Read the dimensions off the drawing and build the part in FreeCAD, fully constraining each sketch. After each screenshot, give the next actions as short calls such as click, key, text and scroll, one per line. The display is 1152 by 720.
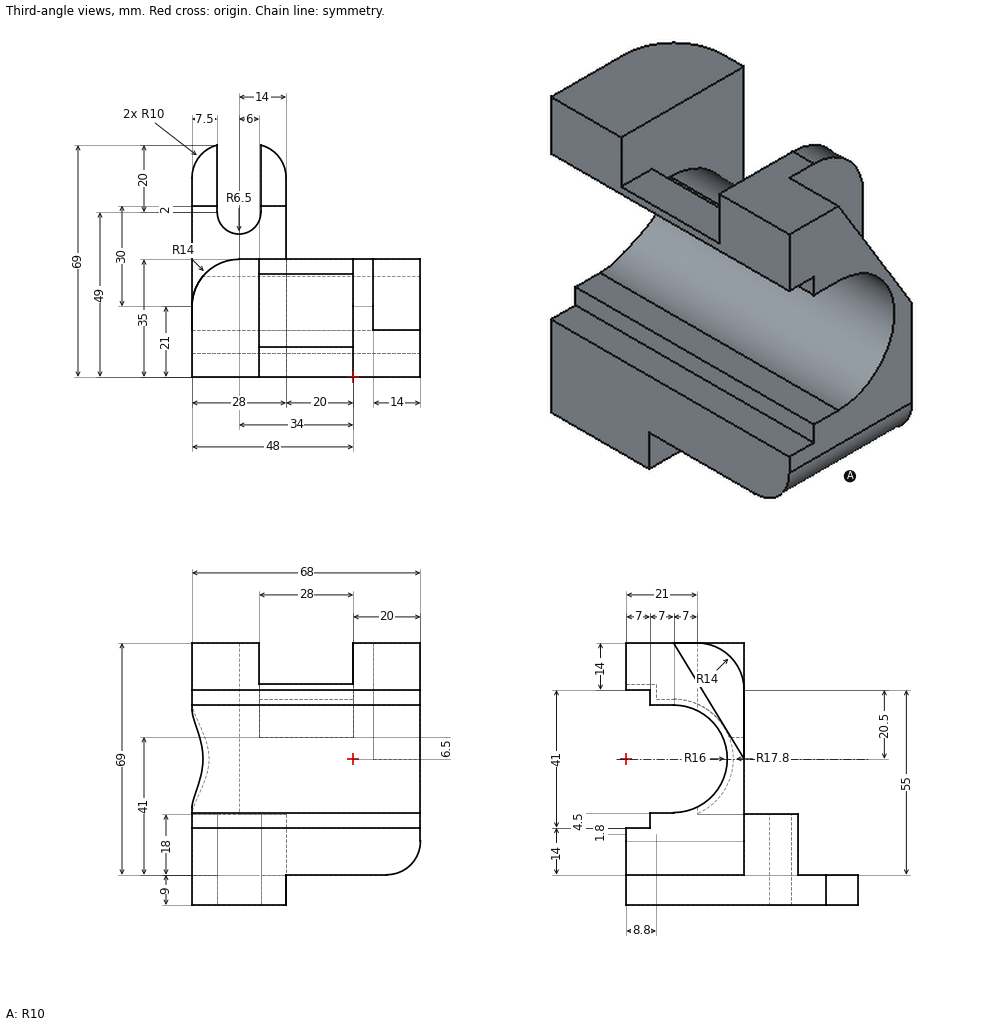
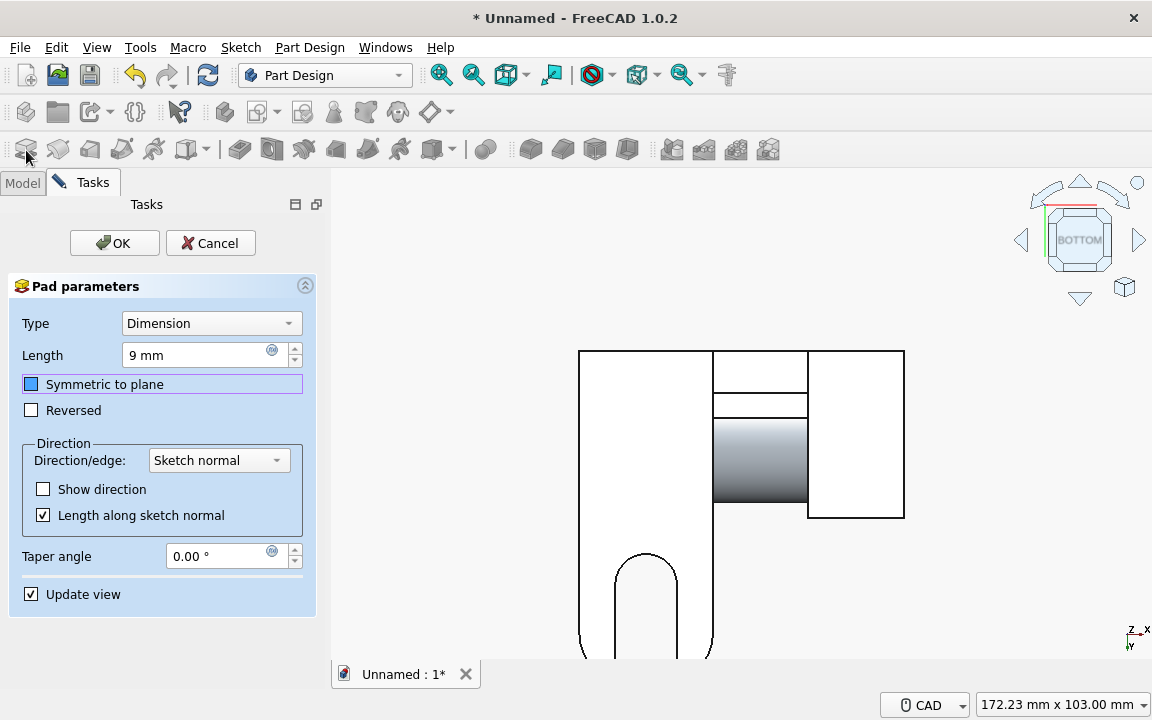
click(115, 243)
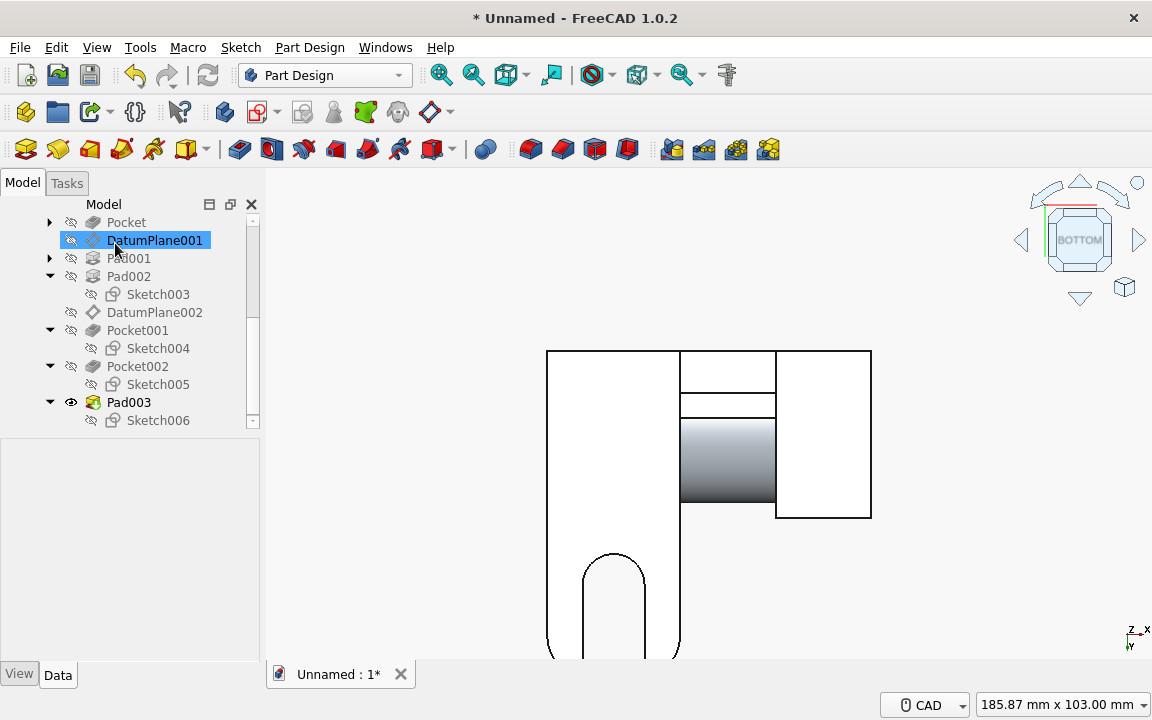
click(442, 76)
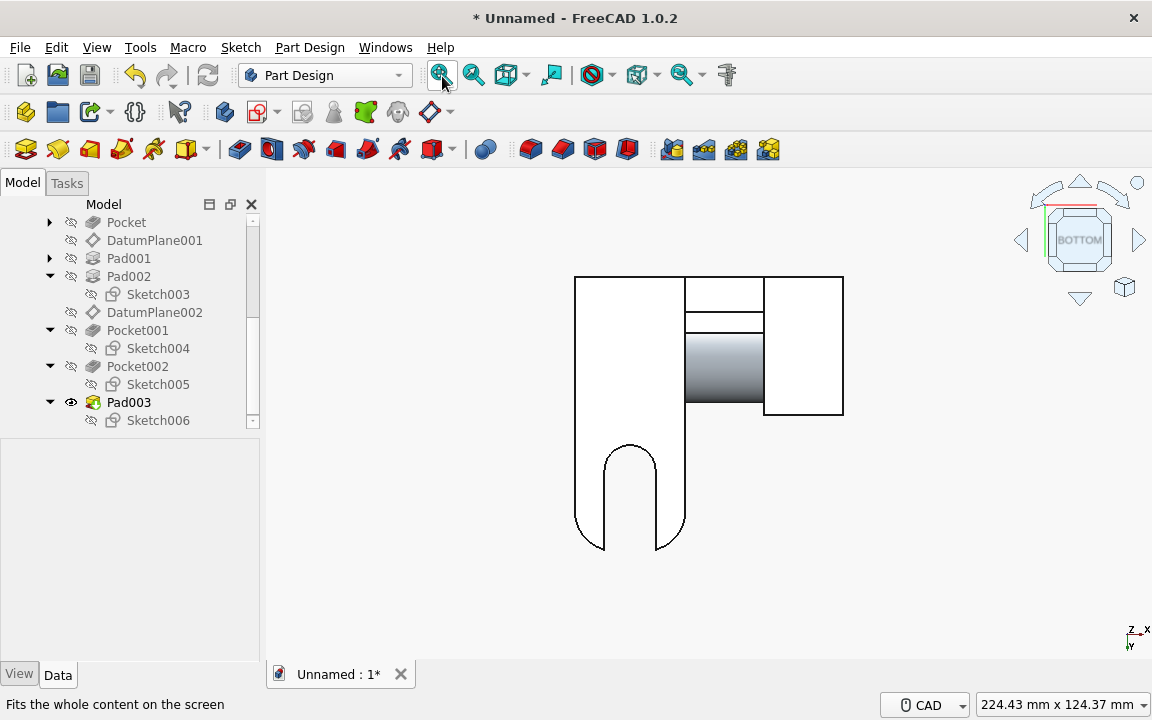
key(4)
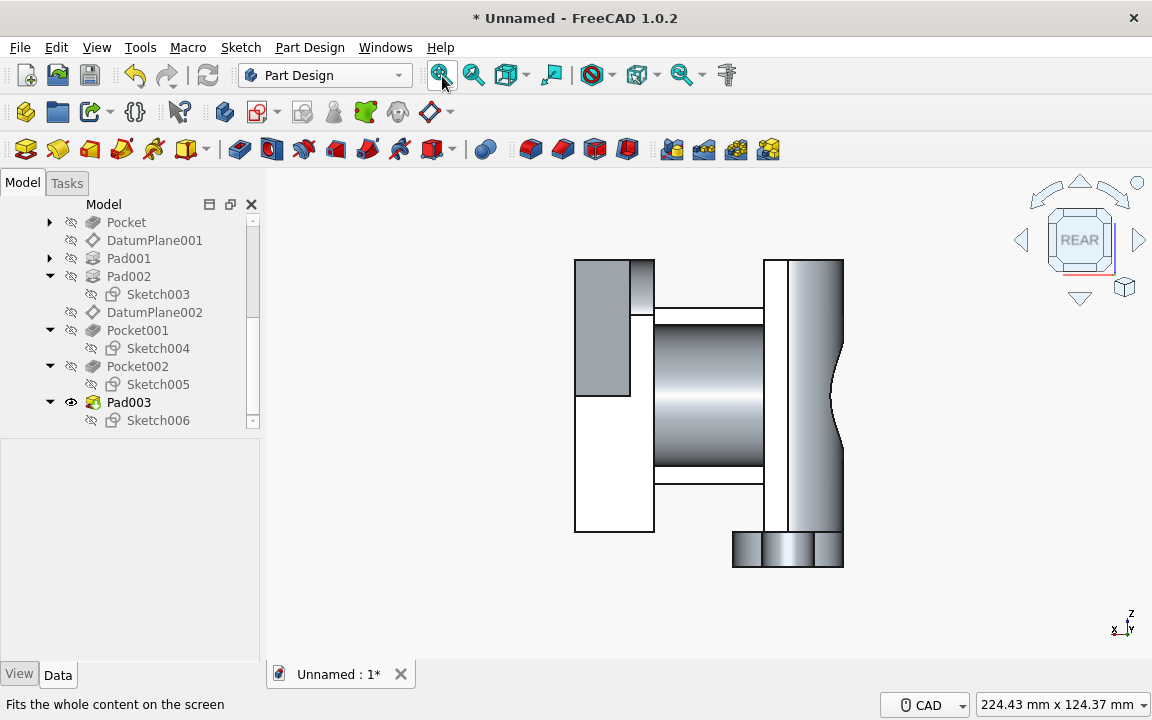
click(614, 484)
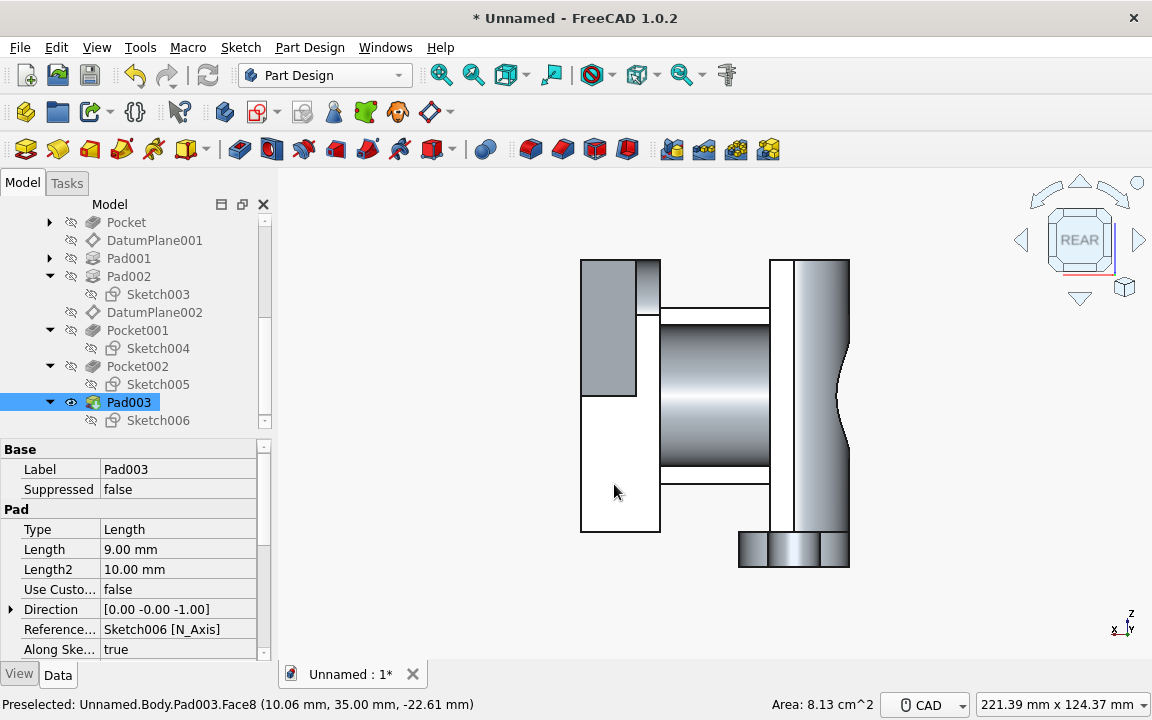
click(258, 112)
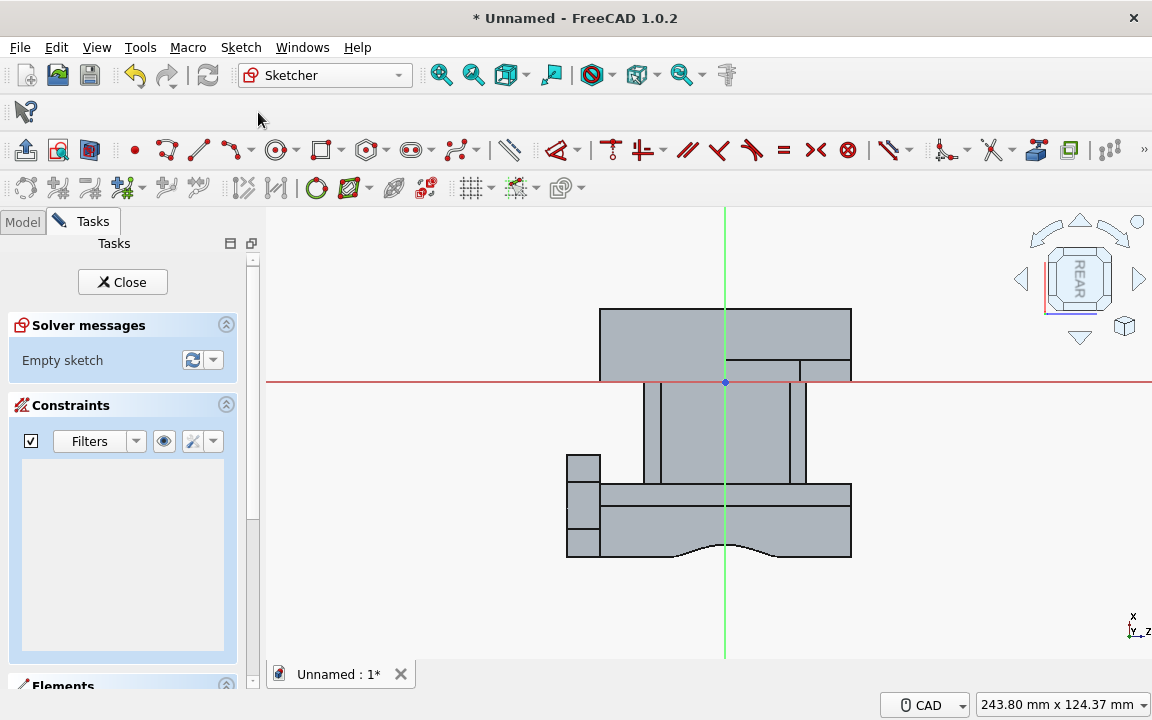
scroll(694, 433, up, 5)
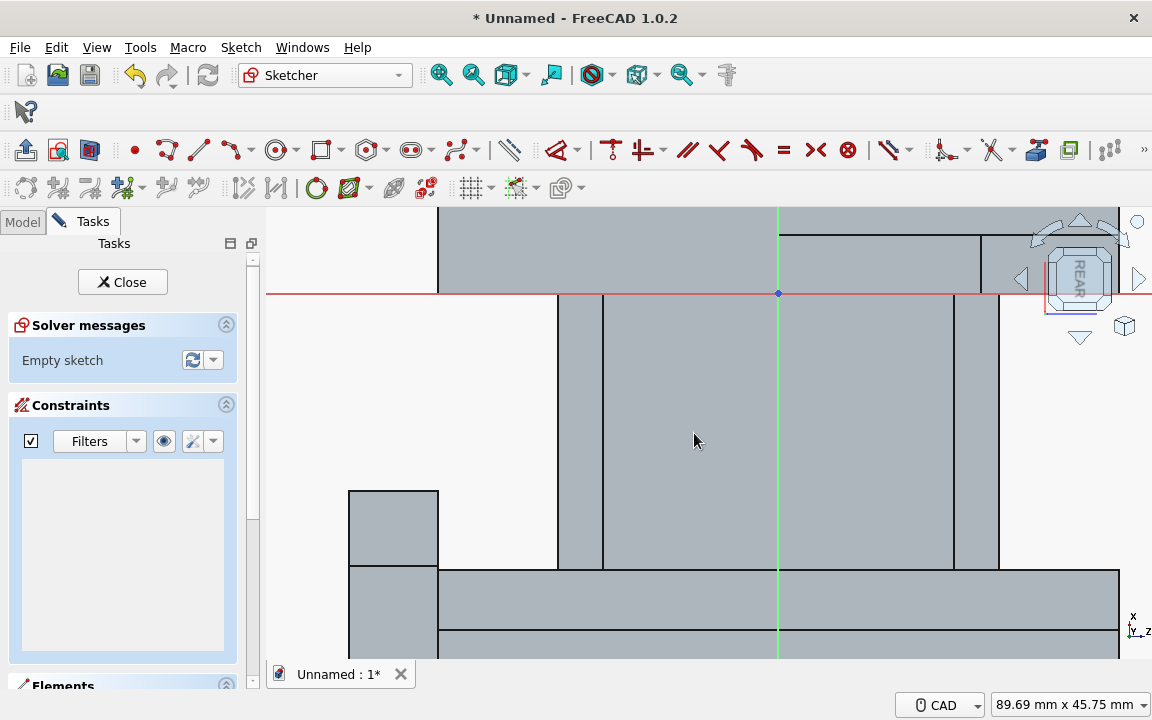
click(322, 150)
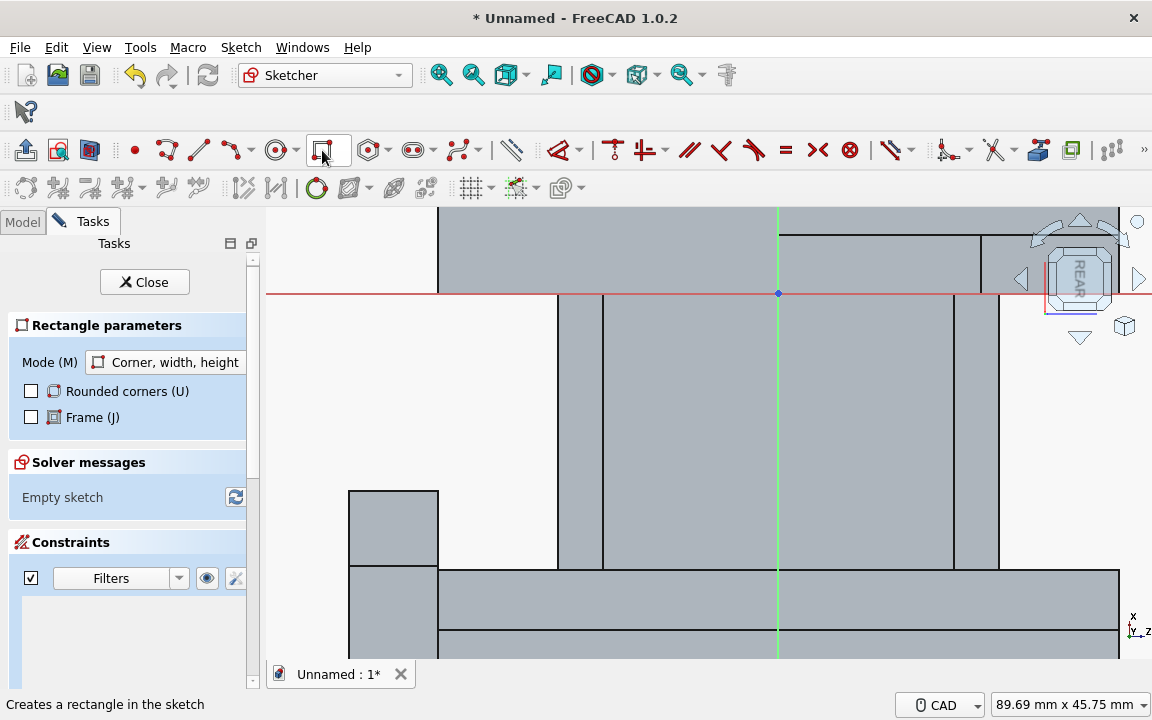
click(438, 294)
move(843, 570)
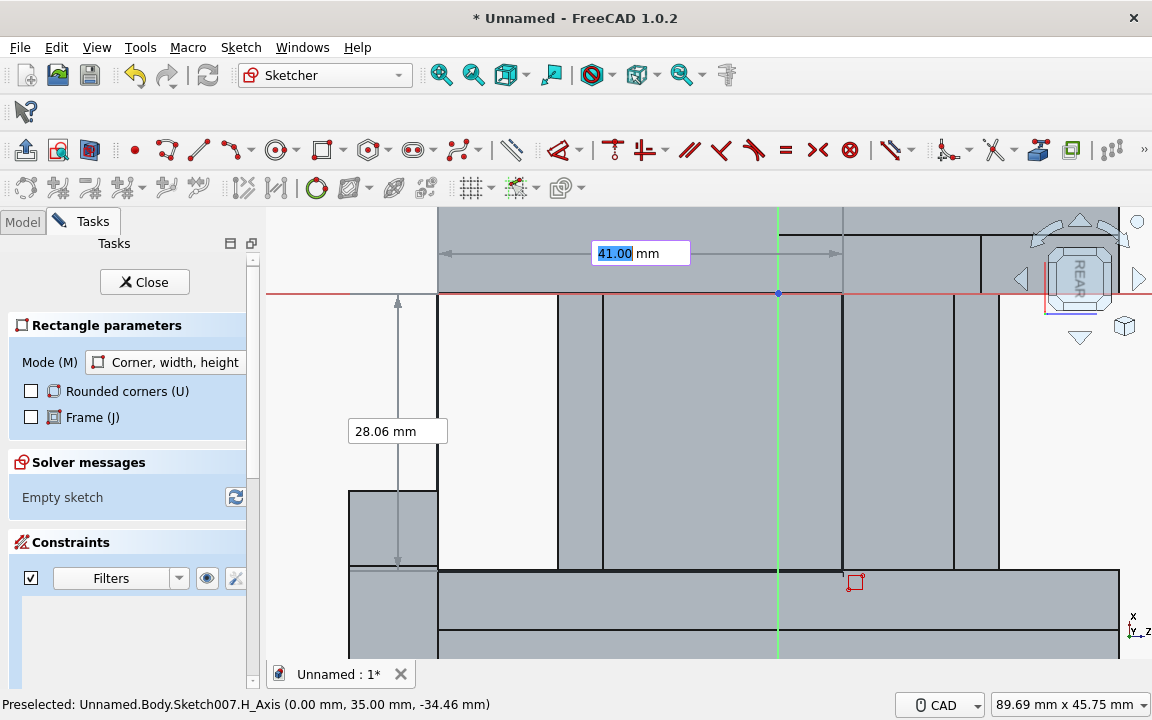
text(41)
key(Tab)
text(28)
key(Return)
key(Escape)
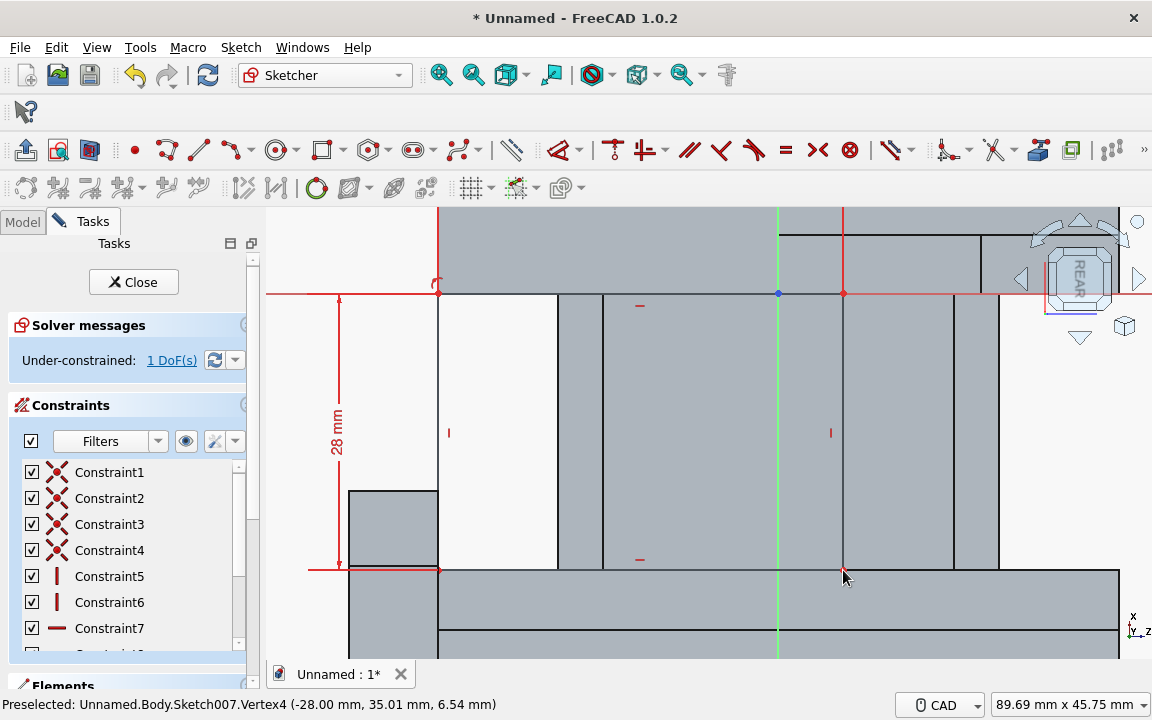
click(558, 150)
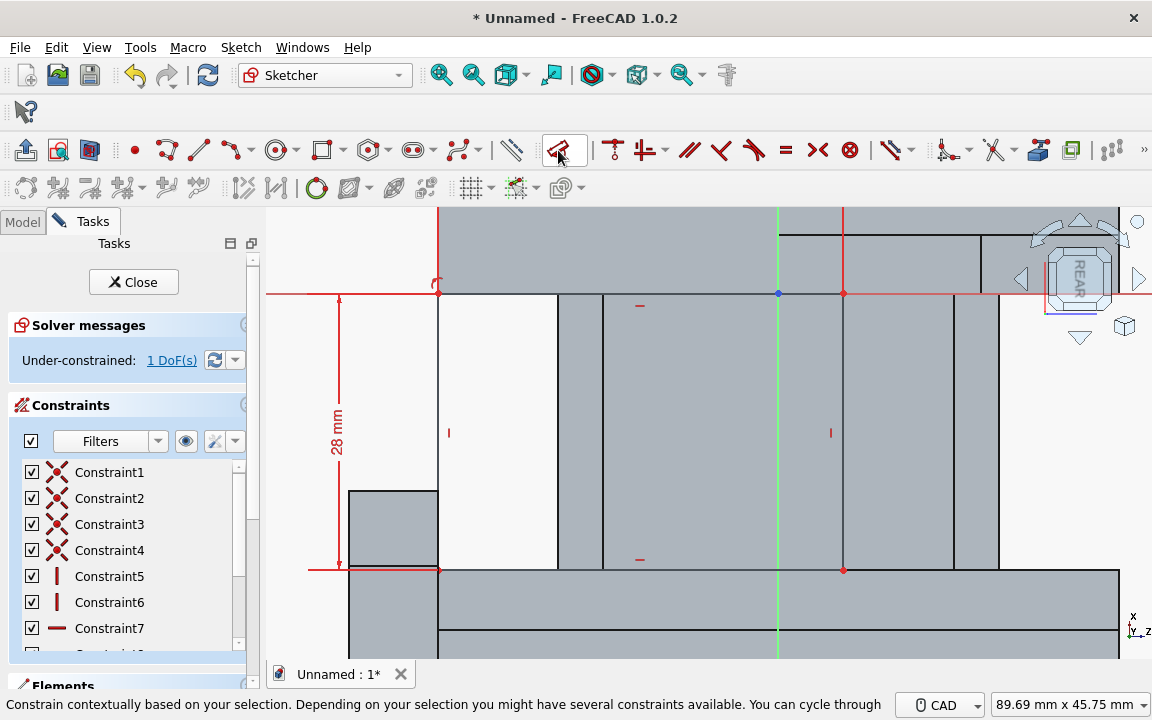
click(843, 570)
click(811, 604)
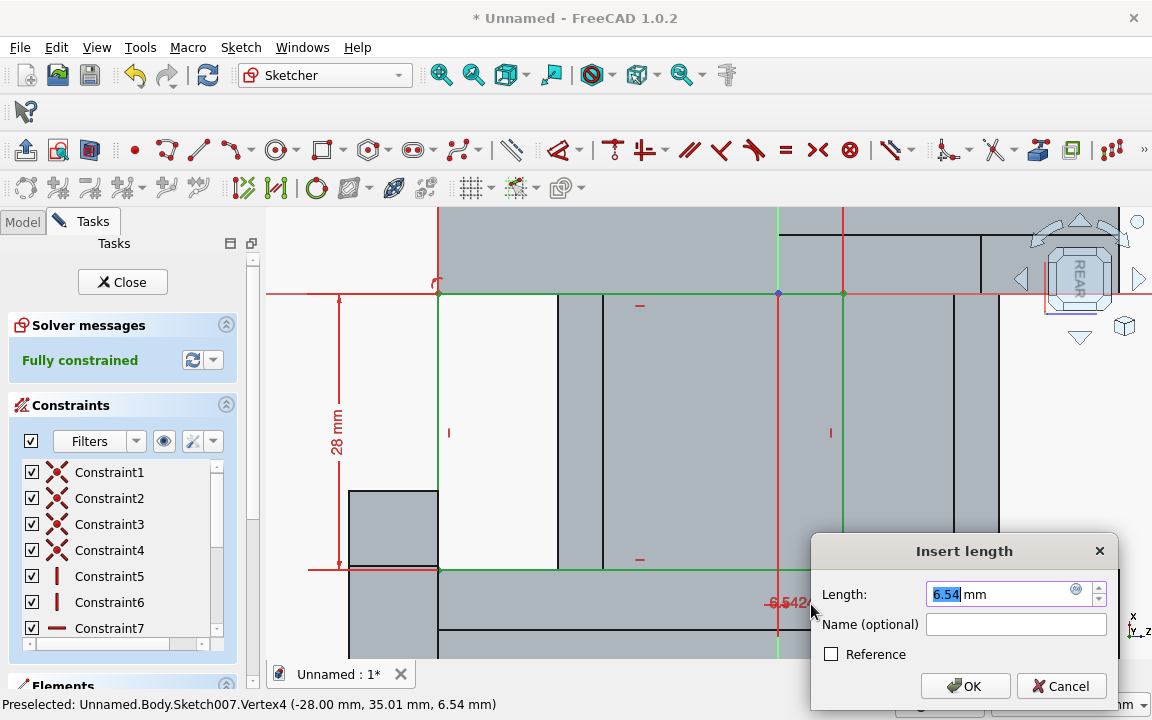
text(6.5)
key(Return)
key(Escape)